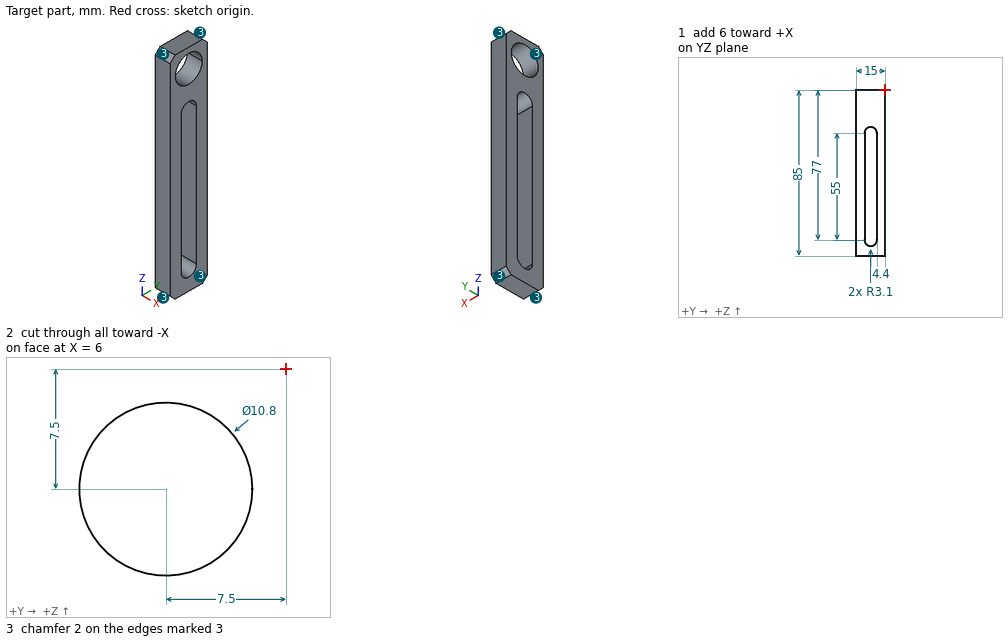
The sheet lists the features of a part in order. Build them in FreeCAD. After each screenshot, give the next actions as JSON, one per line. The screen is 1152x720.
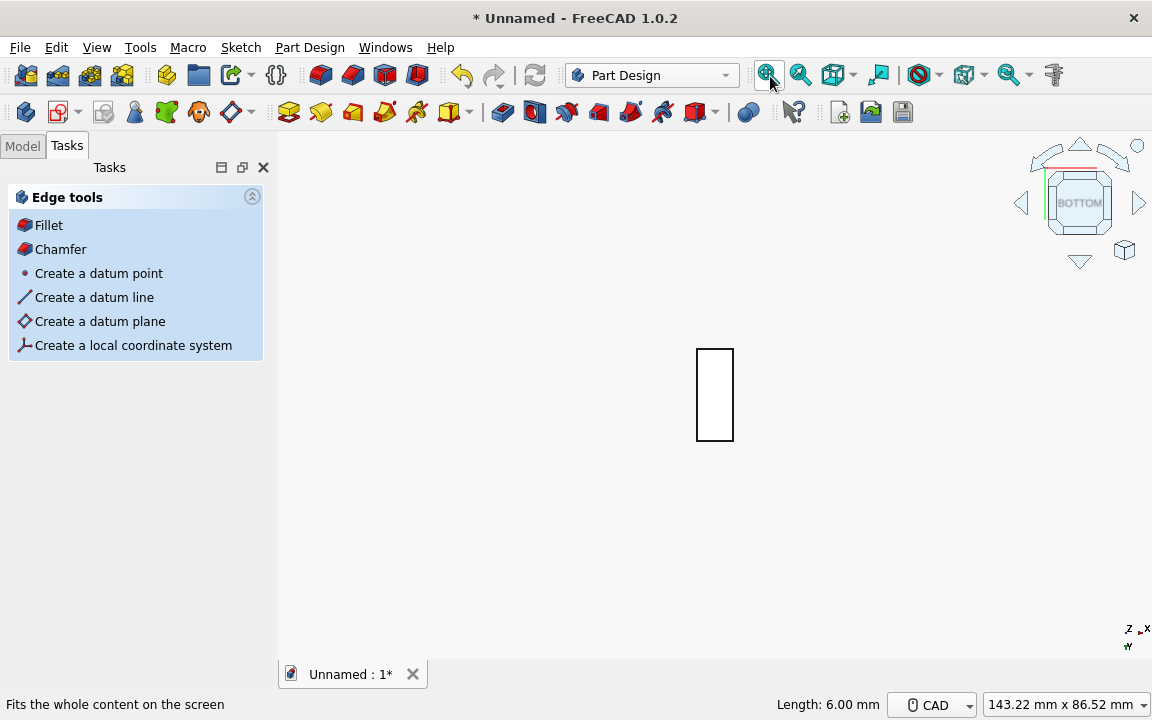
{"action": "left_click", "coordinate": [770, 76]}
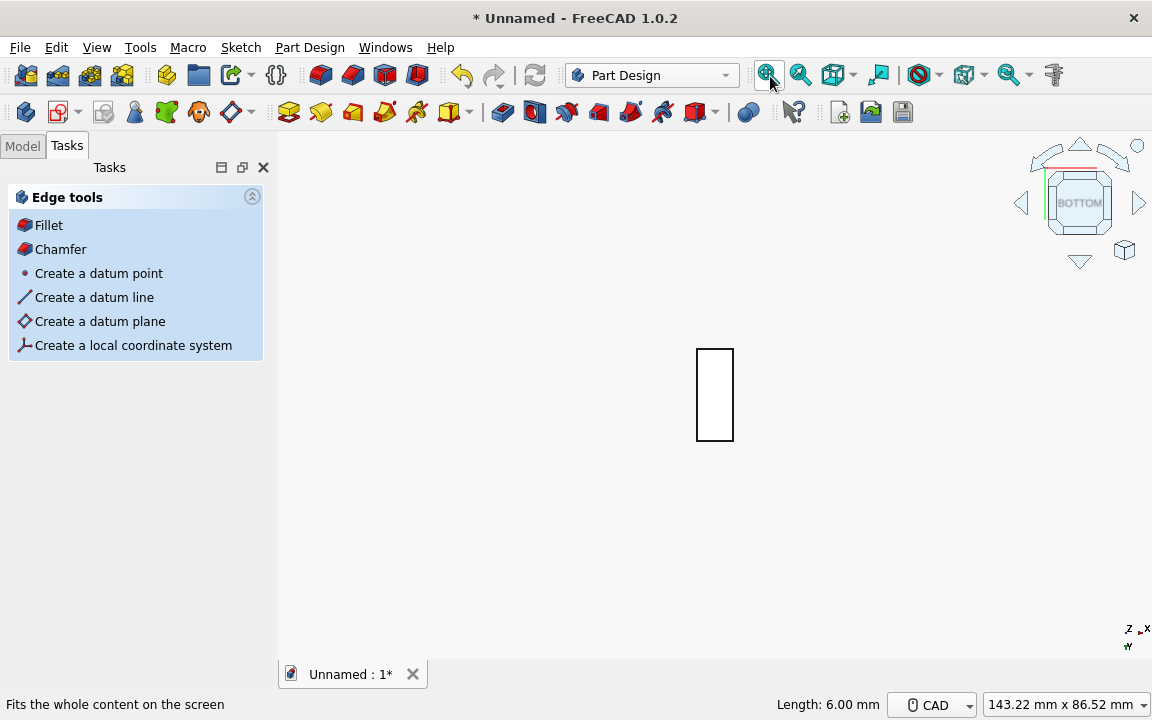
{"action": "left_click", "coordinate": [715, 440], "text": "ctrl"}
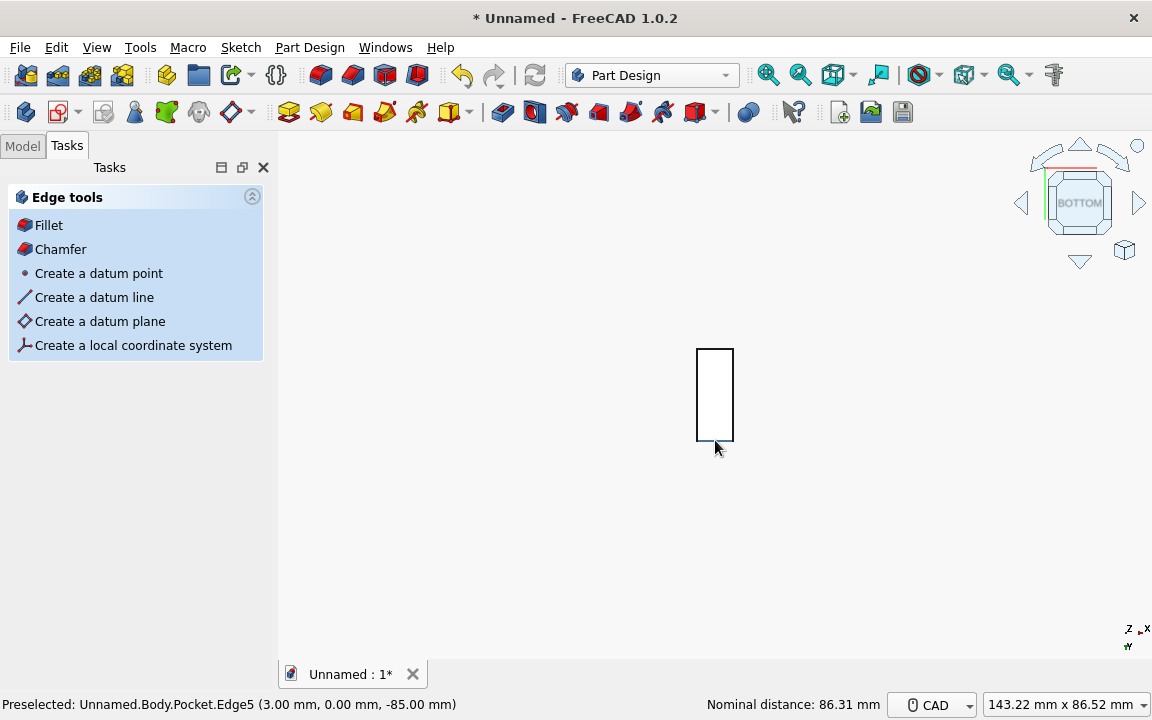
{"action": "left_click", "coordinate": [715, 348], "text": "ctrl"}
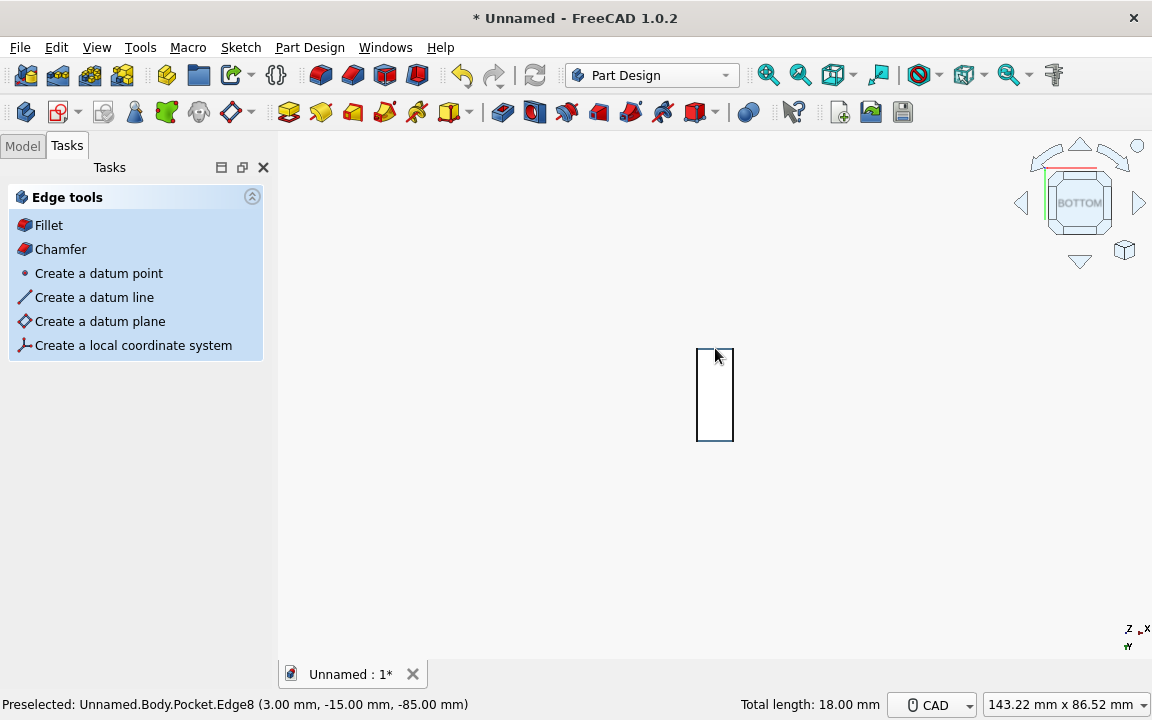
{"action": "key", "text": "4"}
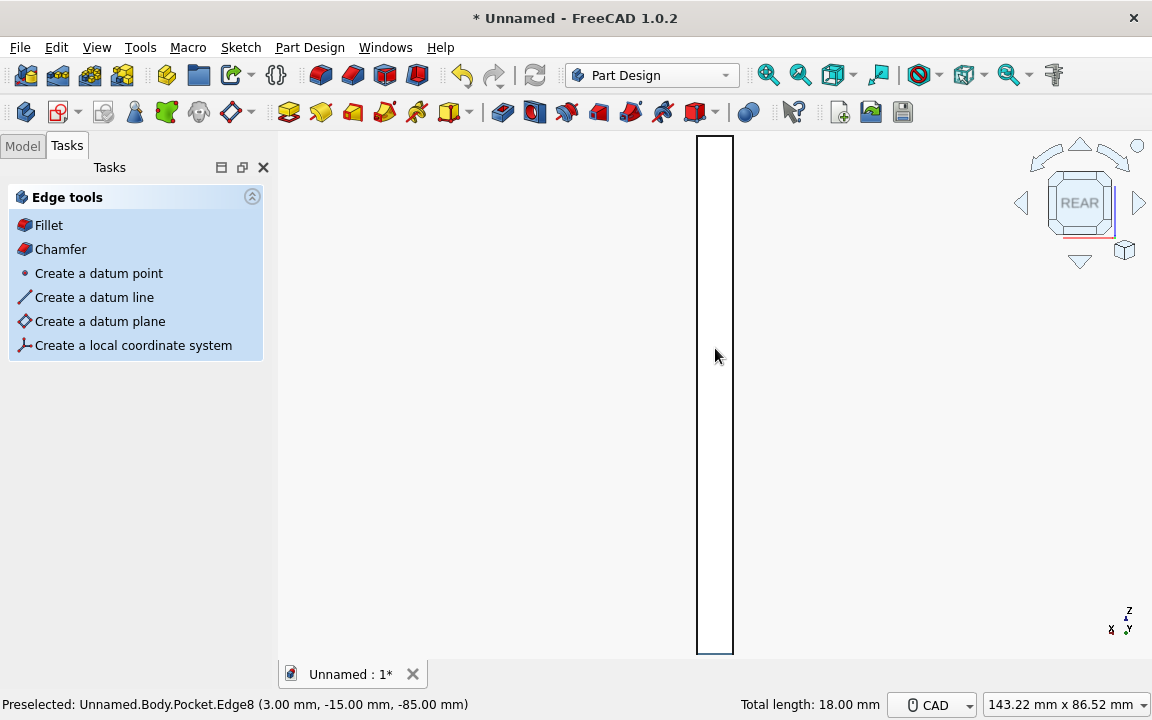
{"action": "key", "text": "6"}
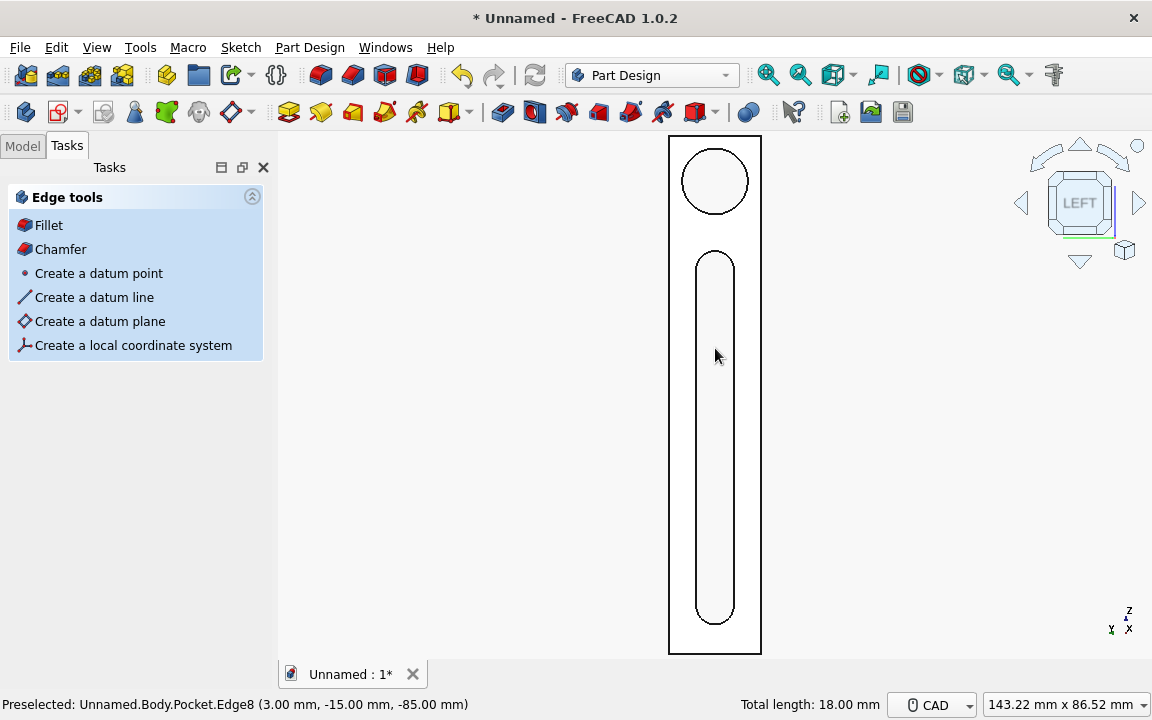
{"action": "key", "text": "v 3"}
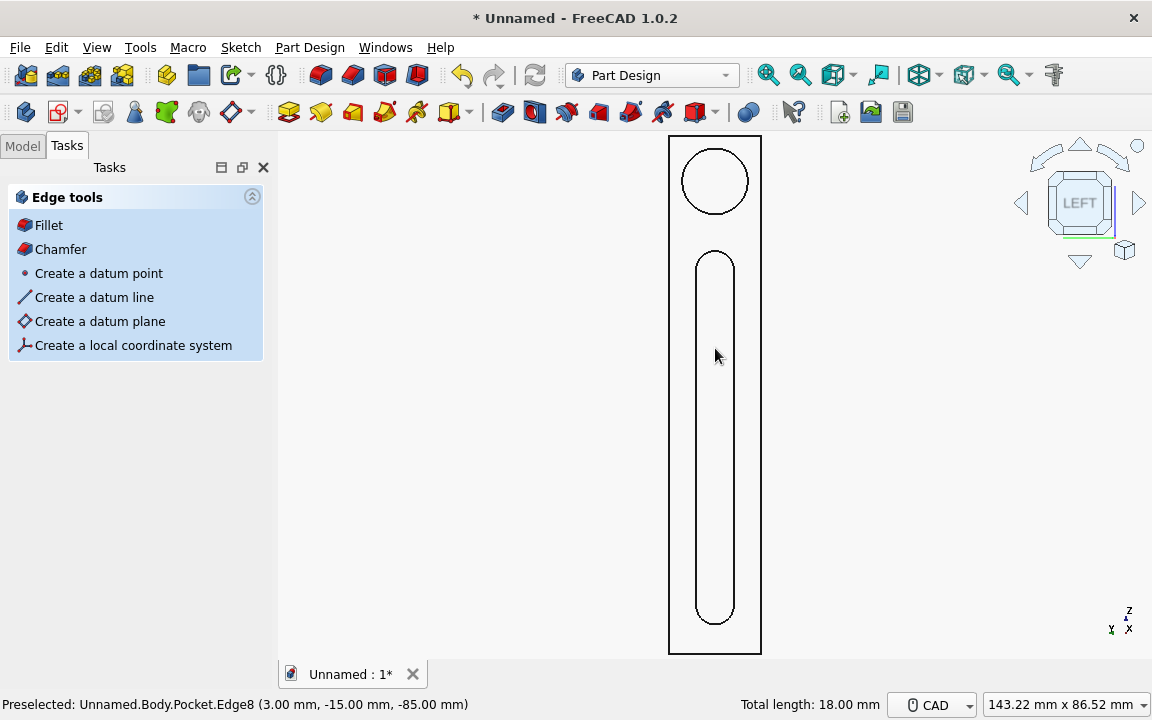
{"action": "key", "text": "0"}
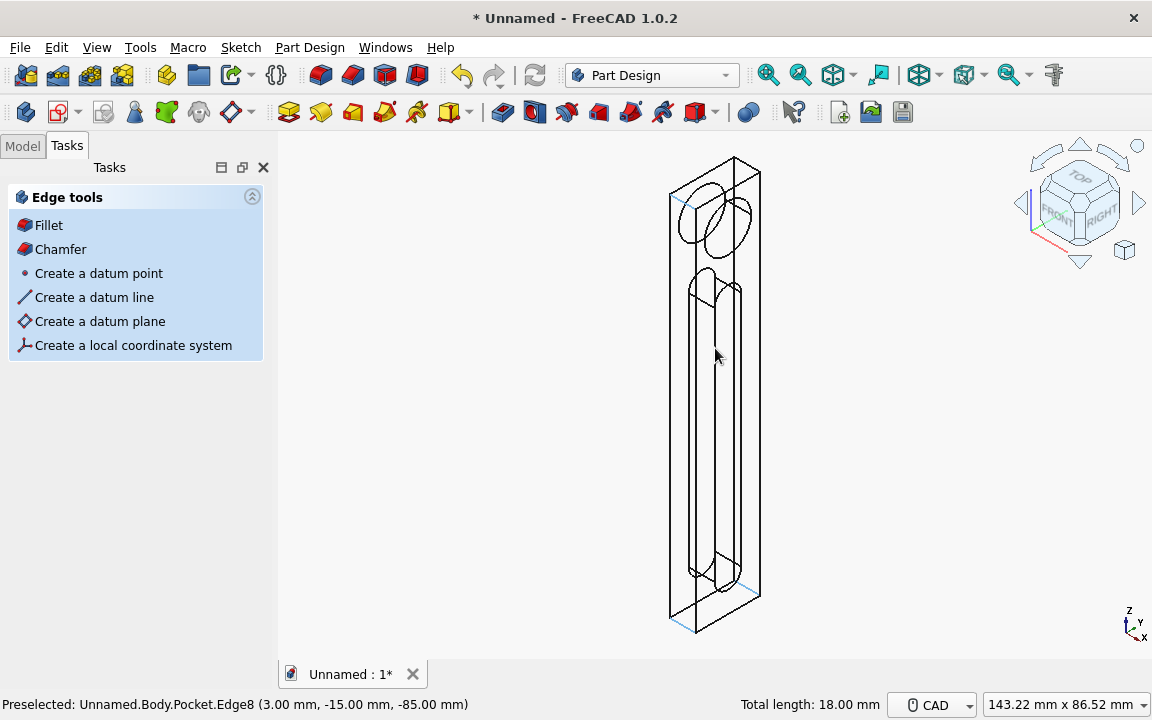
{"action": "left_click", "coordinate": [747, 164], "text": "ctrl"}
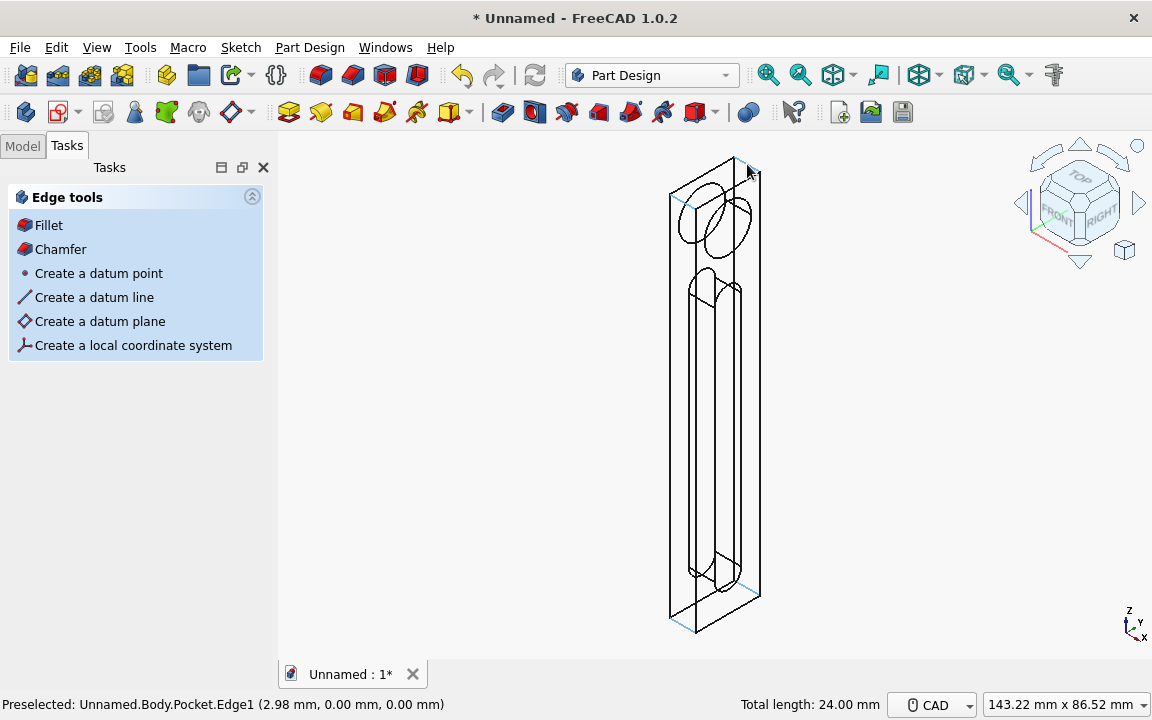
{"action": "key", "text": "v 1"}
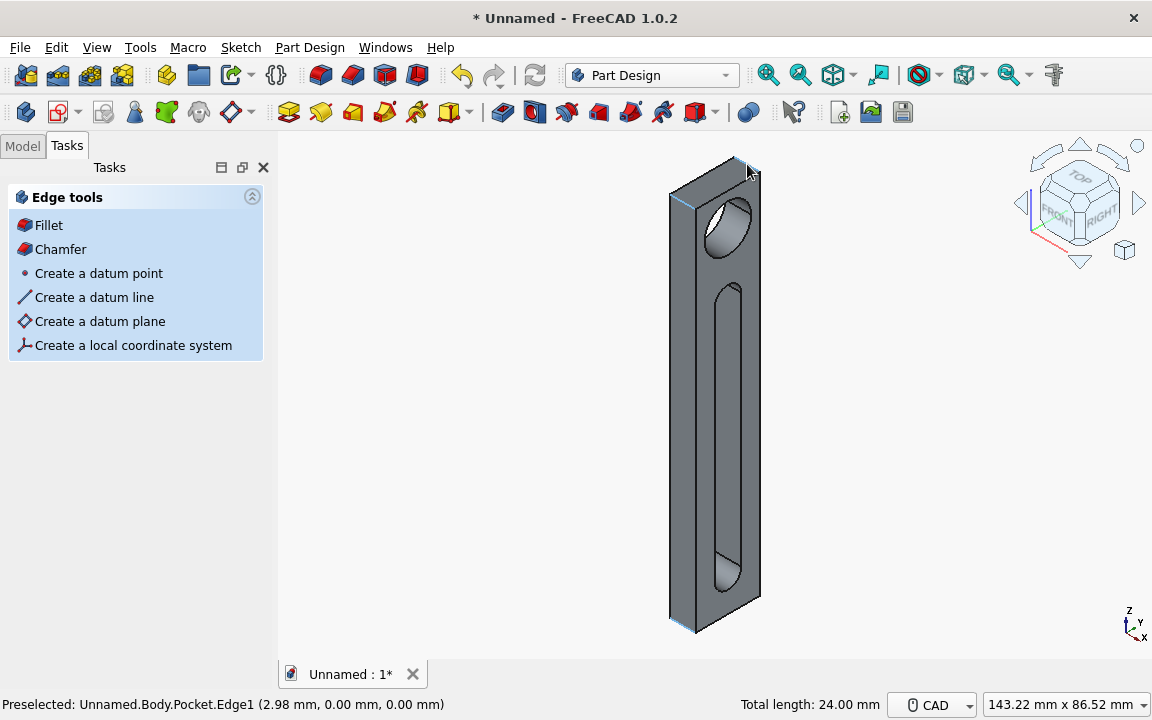
{"action": "left_click", "coordinate": [354, 76]}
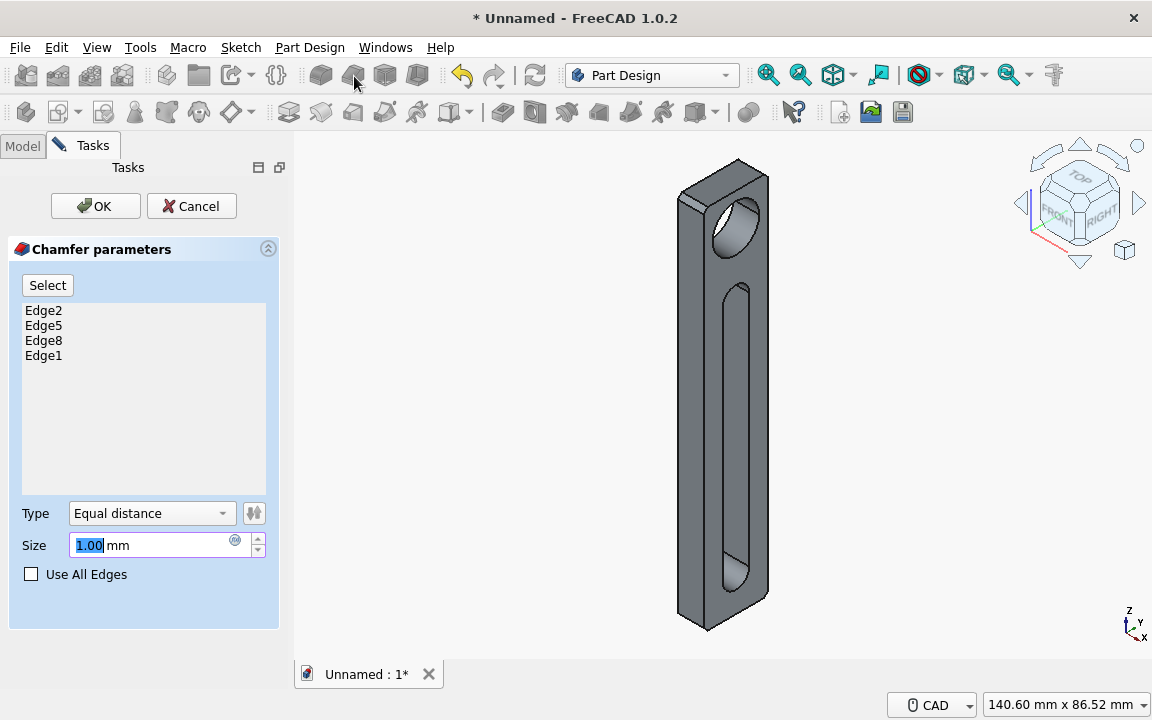
{"action": "type", "text": "2"}
{"action": "key", "text": "Tab"}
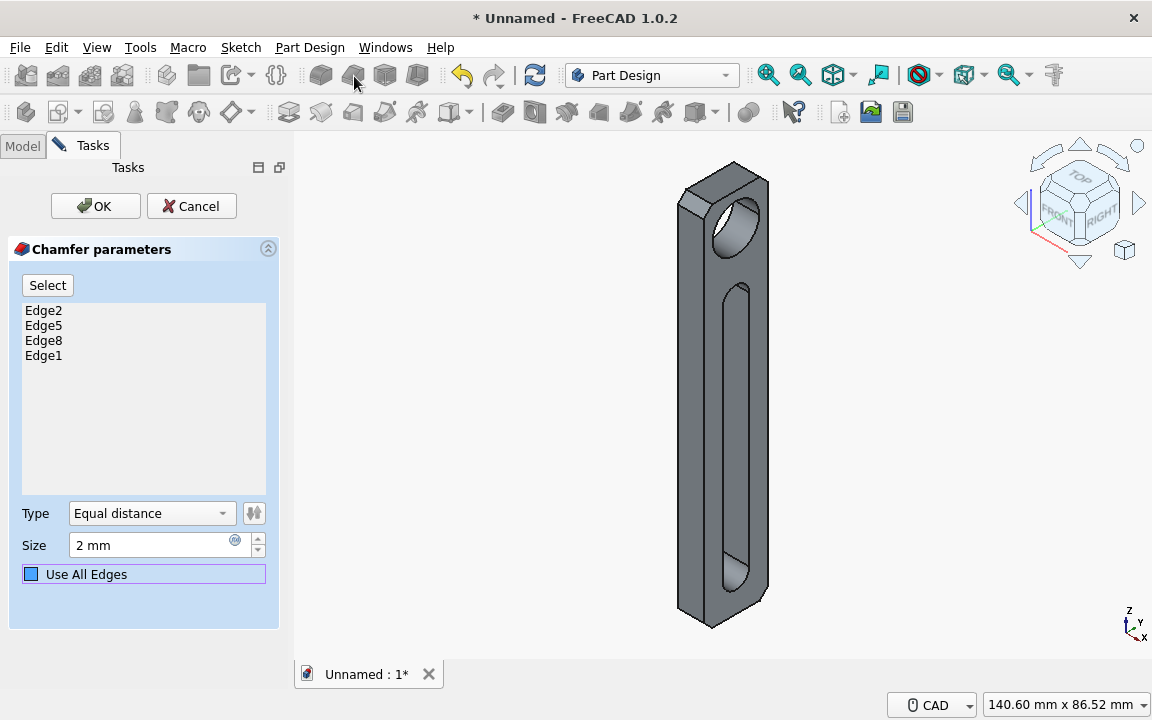
{"action": "left_click", "coordinate": [96, 206]}